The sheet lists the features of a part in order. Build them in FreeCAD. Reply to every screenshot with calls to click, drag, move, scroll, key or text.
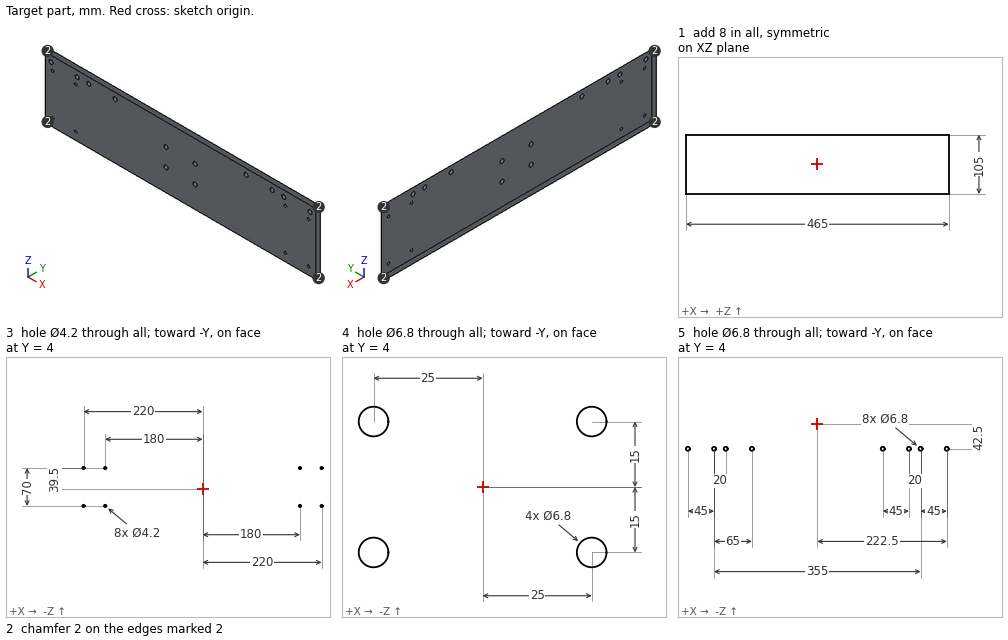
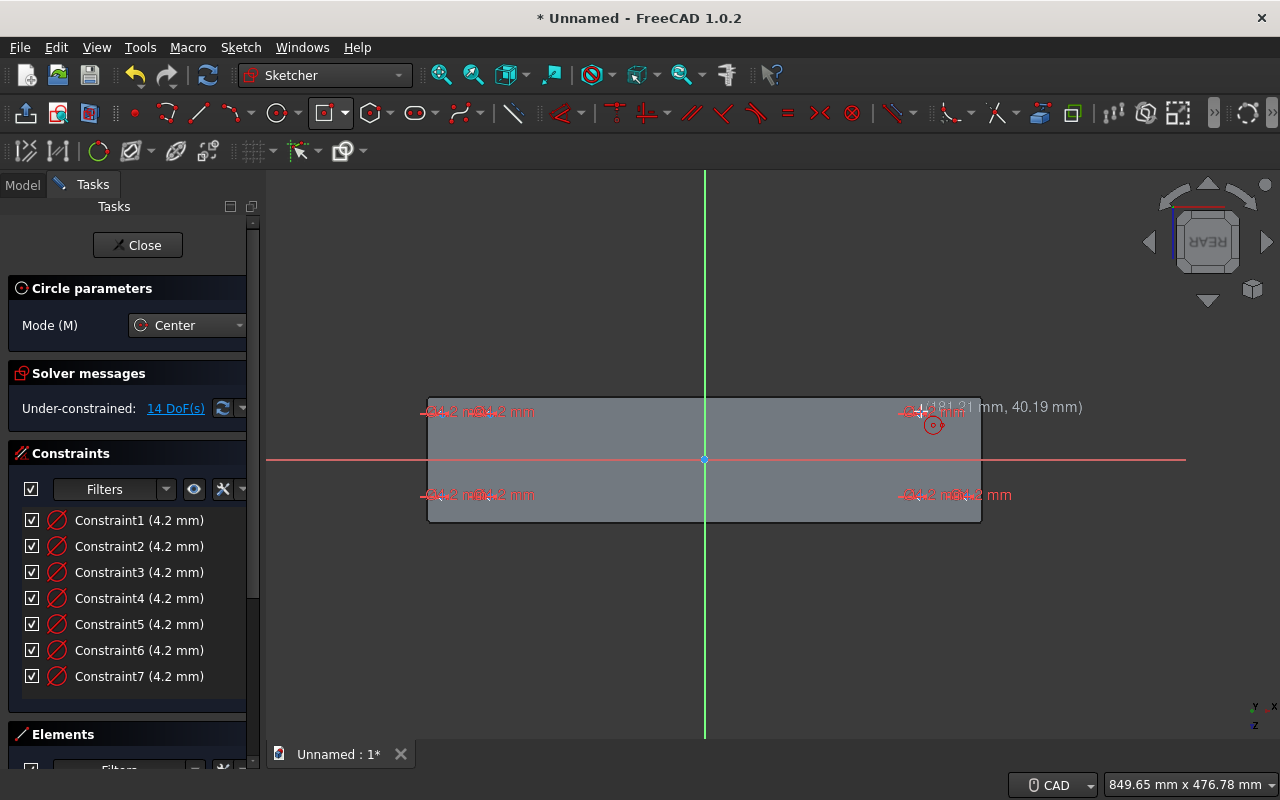
scroll(967, 413, up, 12)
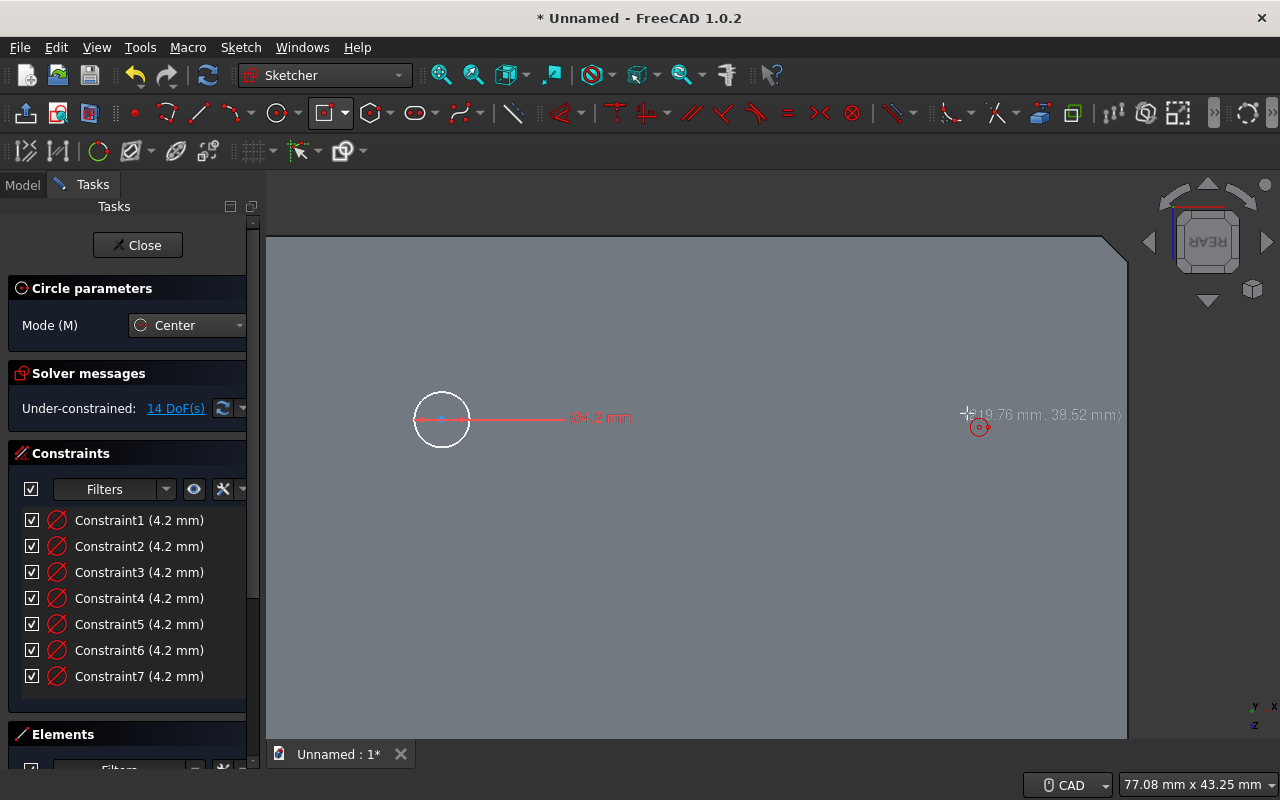
scroll(967, 413, down, 12)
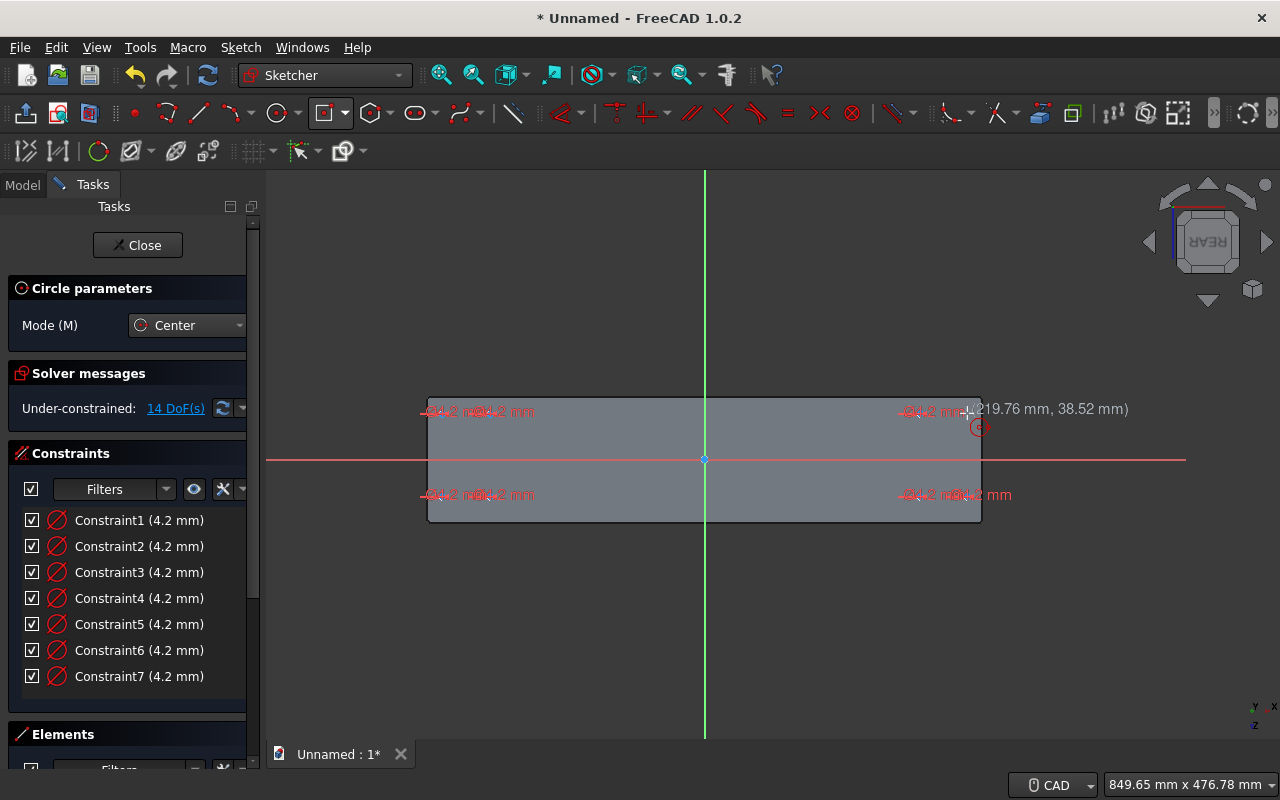
click(967, 413)
move(969, 411)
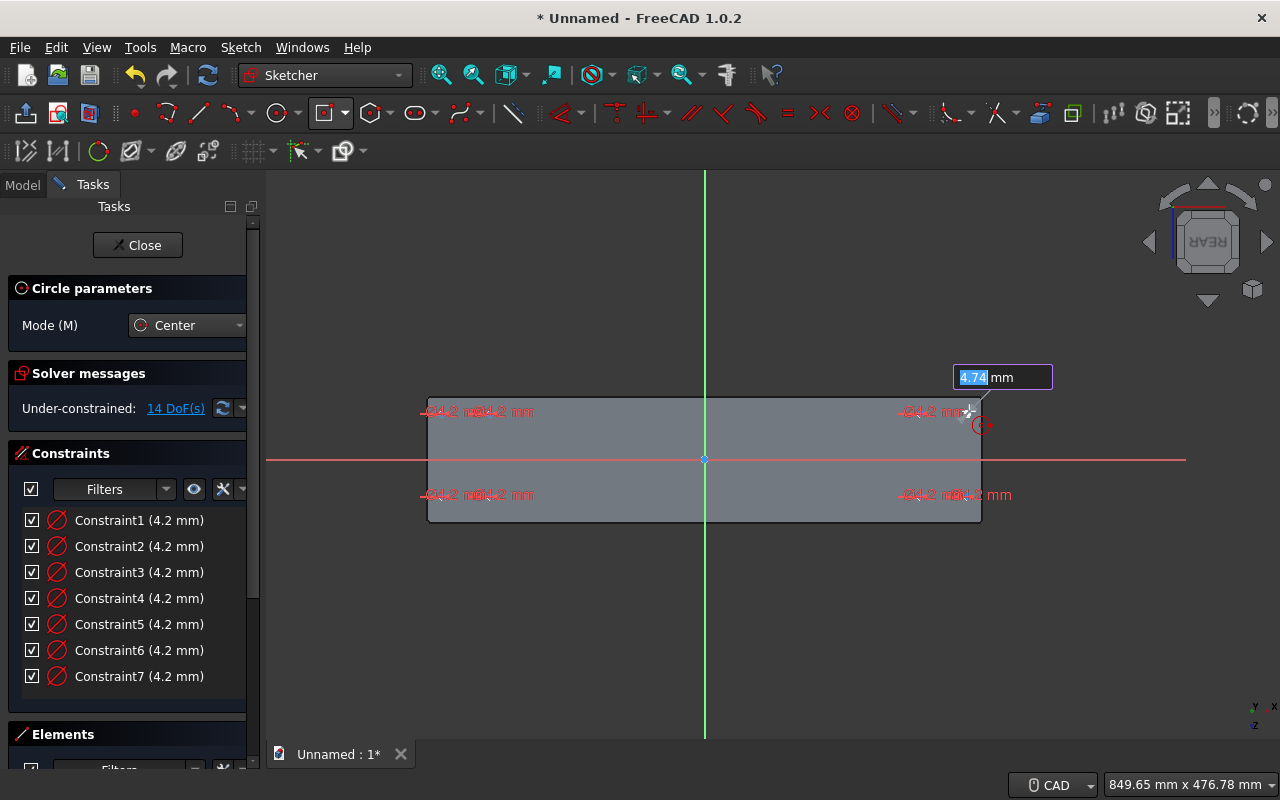
text(4.2)
key(Return)
key(Escape)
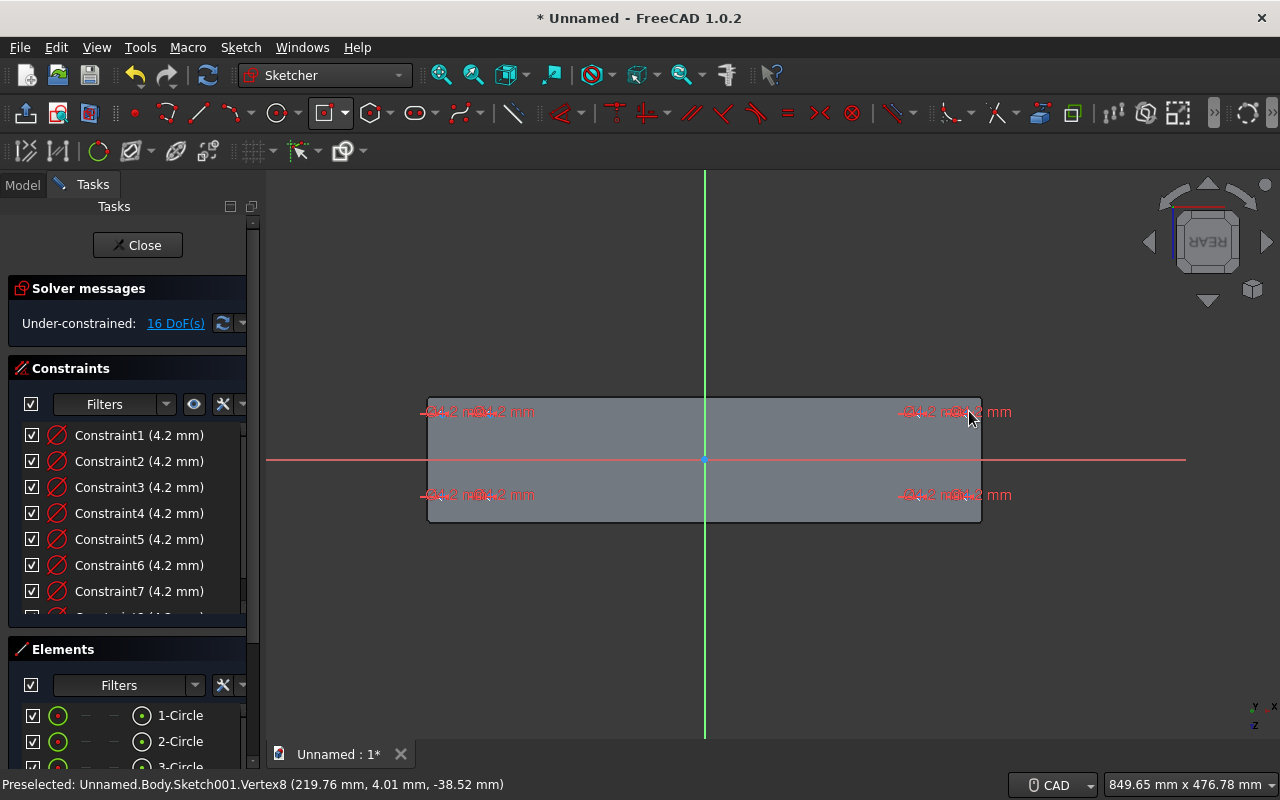
click(442, 414)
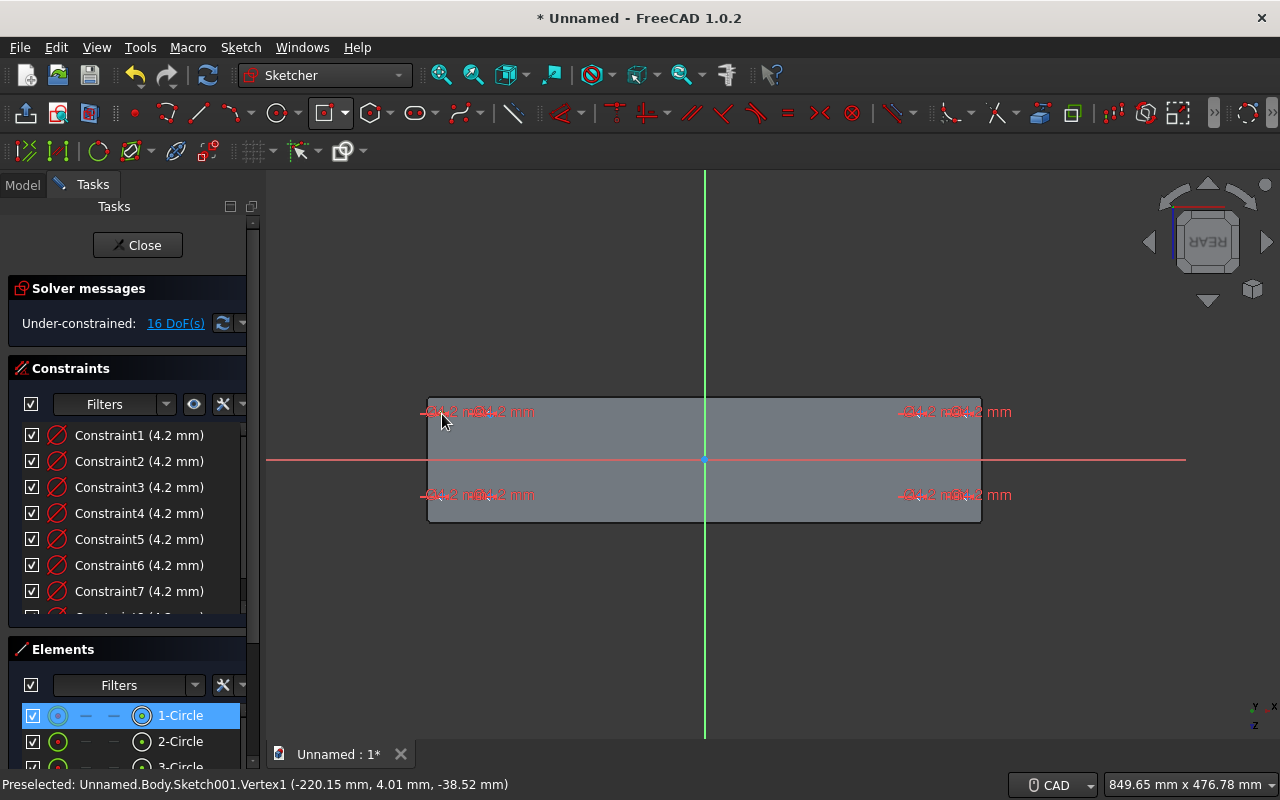
click(490, 414)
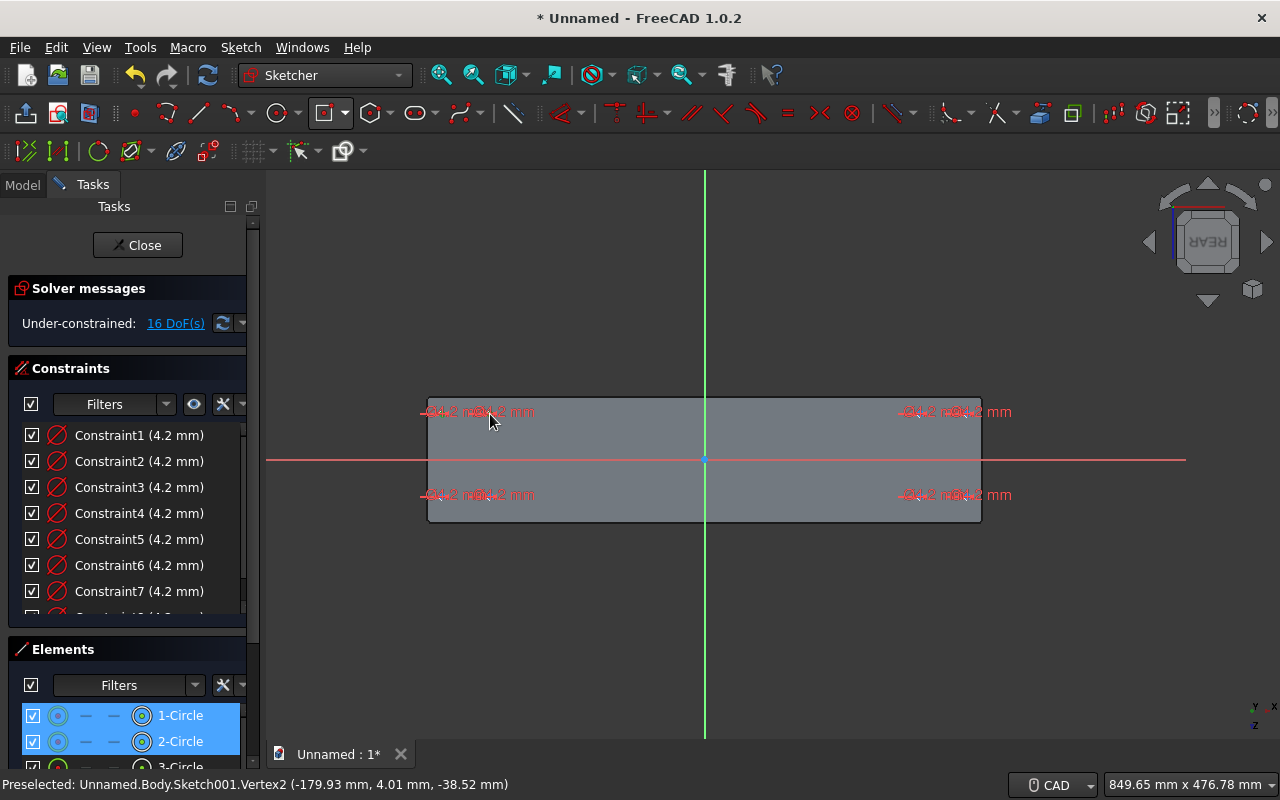
click(670, 114)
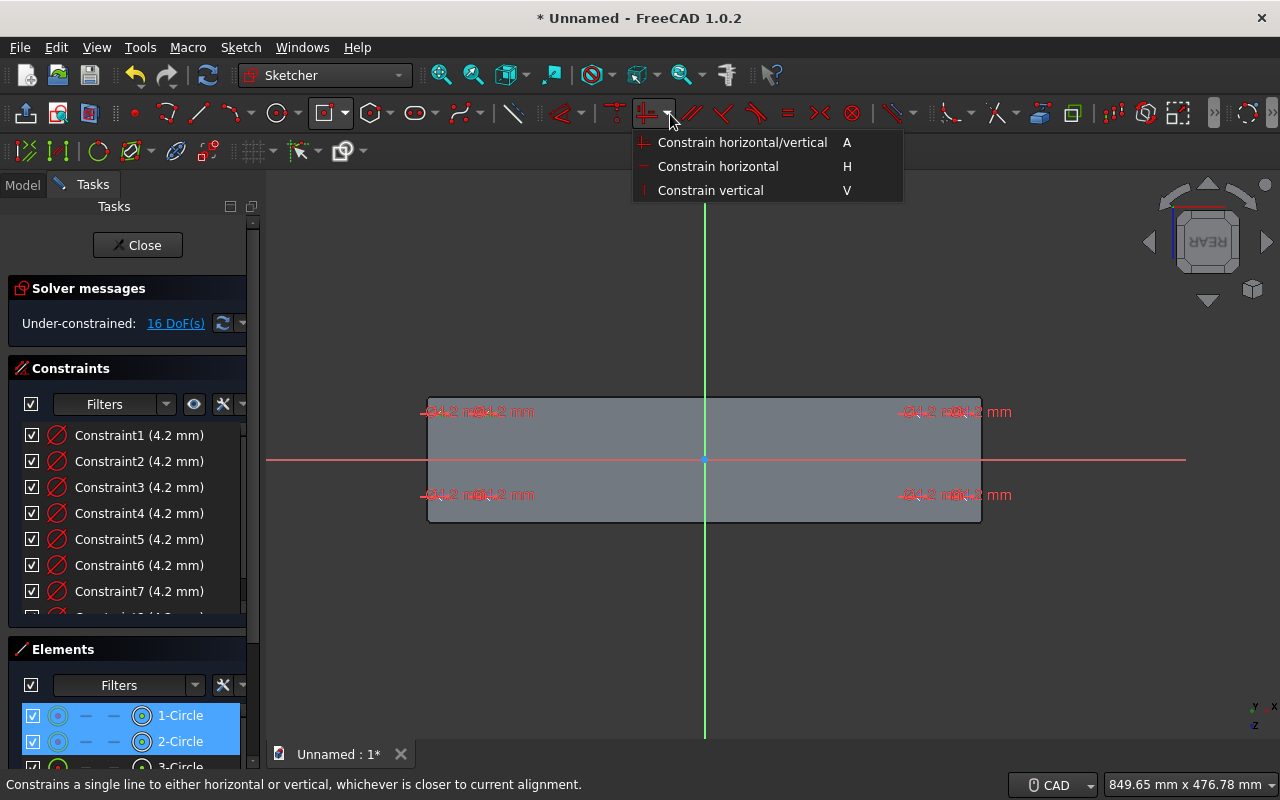
click(768, 166)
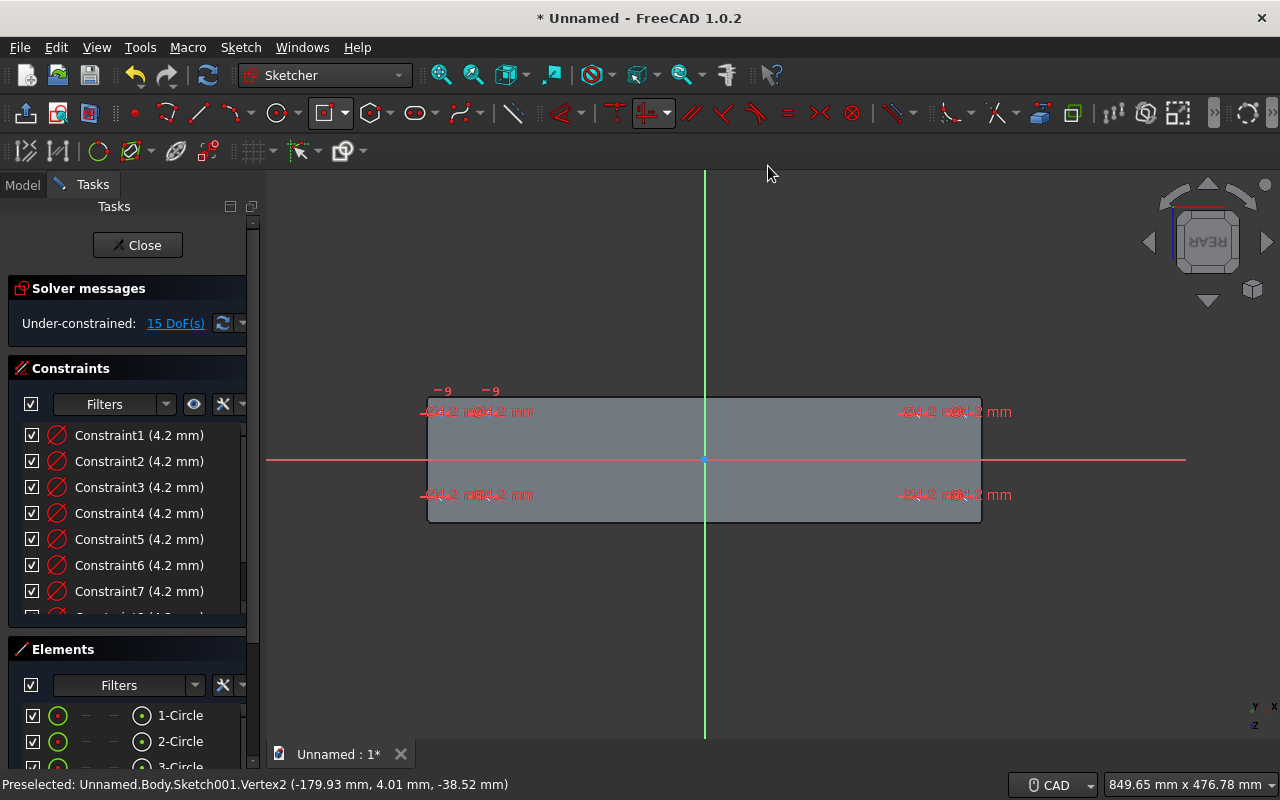
click(490, 414)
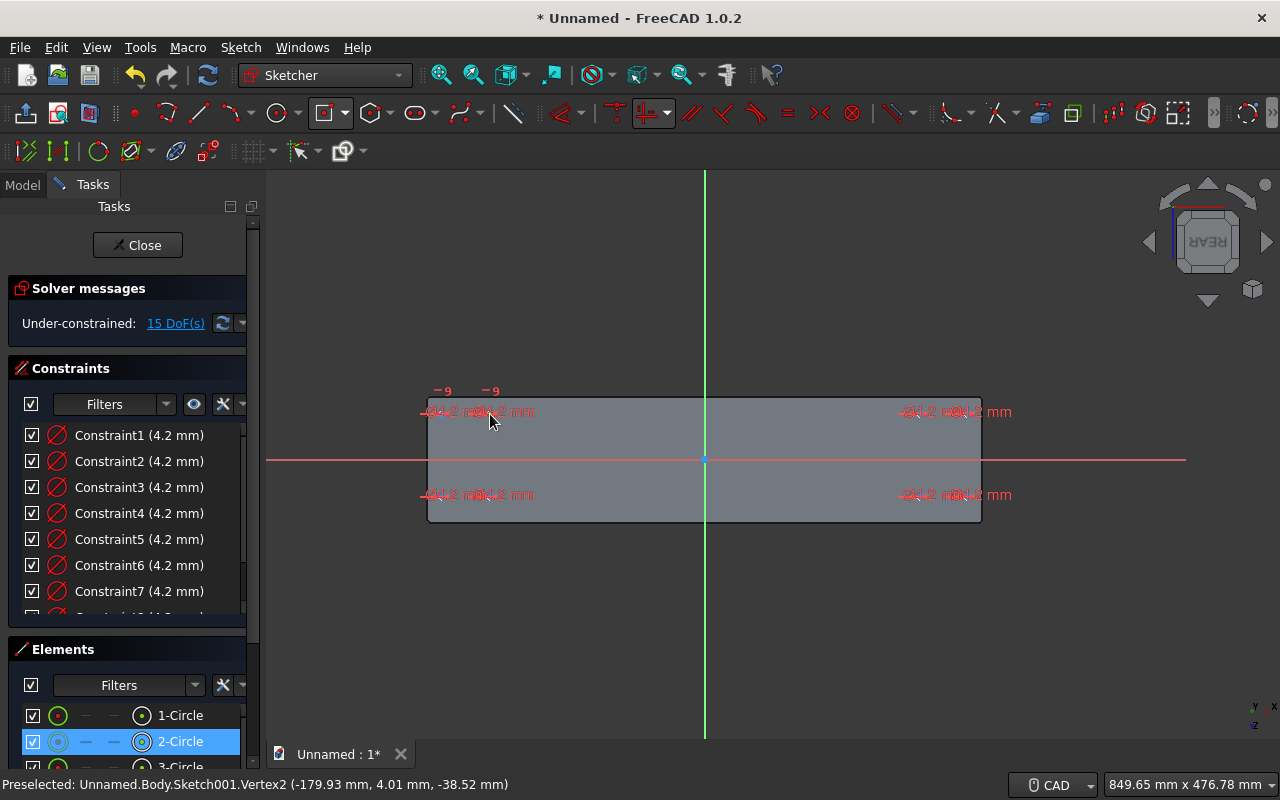
click(490, 497)